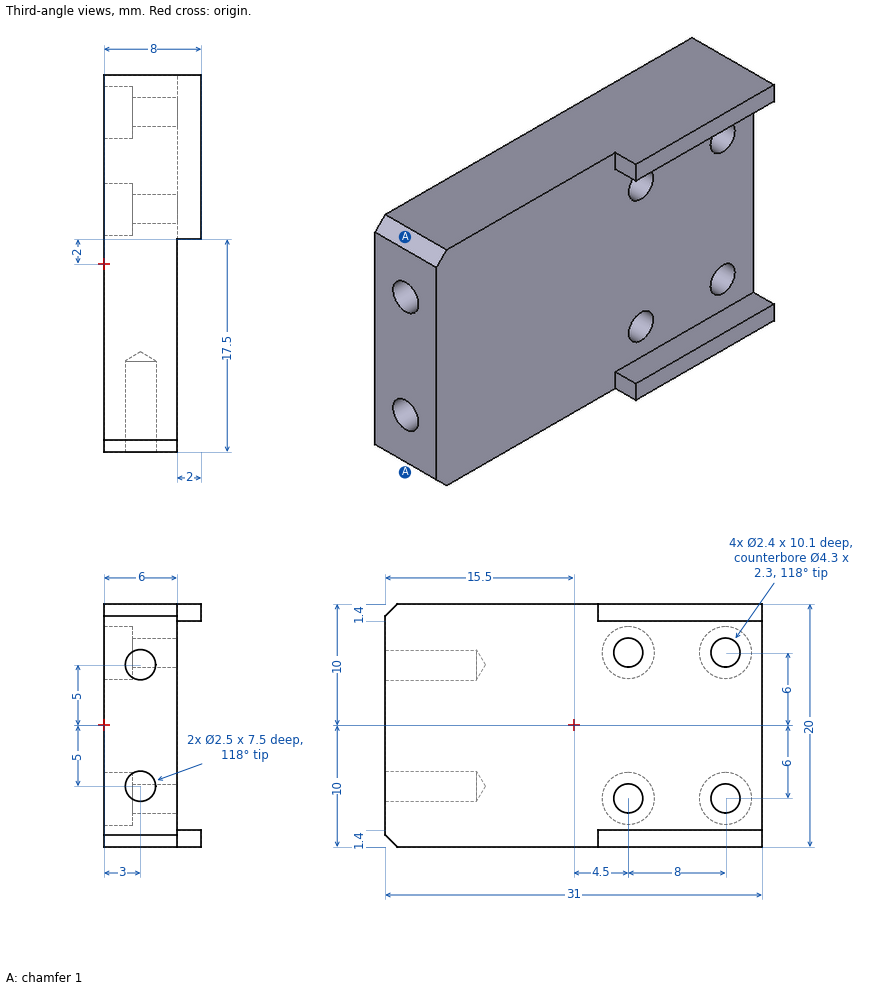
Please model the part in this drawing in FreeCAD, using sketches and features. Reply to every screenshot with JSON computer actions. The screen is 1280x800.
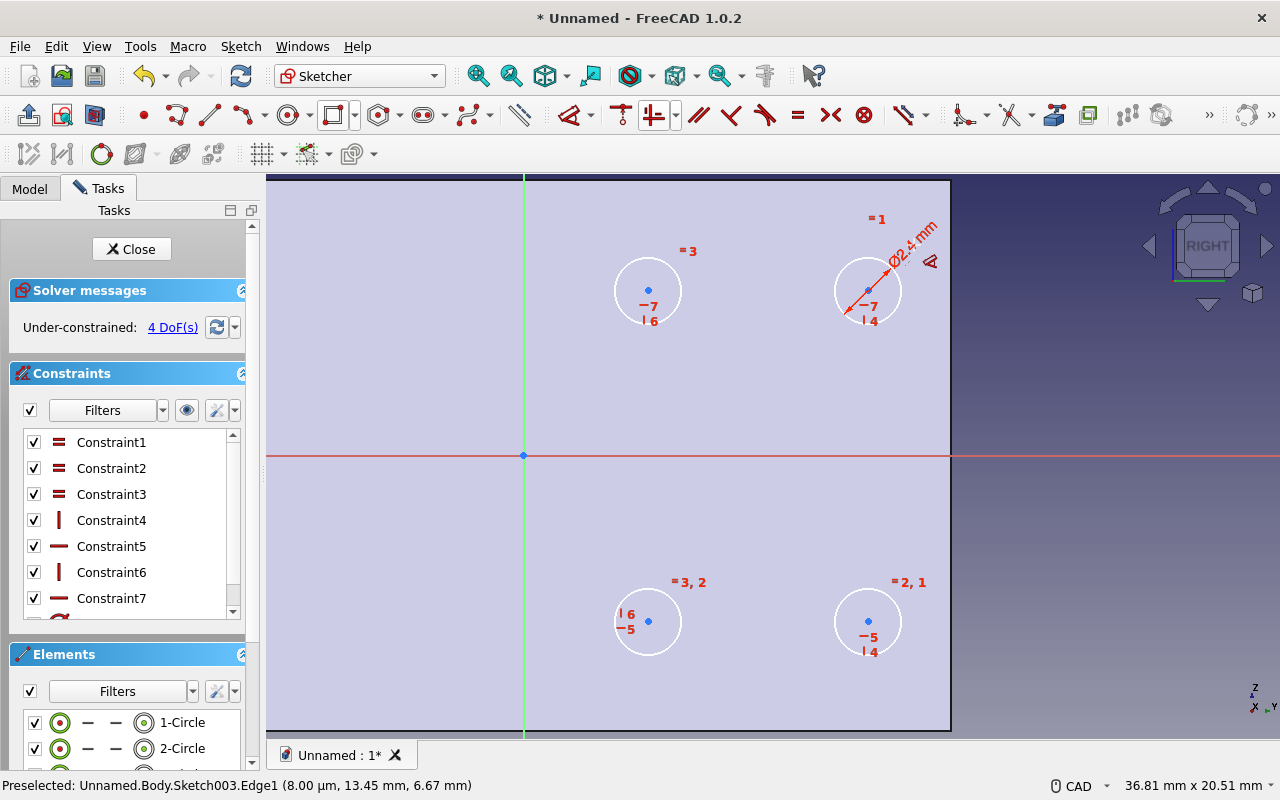
{"action": "left_click", "coordinate": [868, 291]}
{"action": "left_click", "coordinate": [490, 373]}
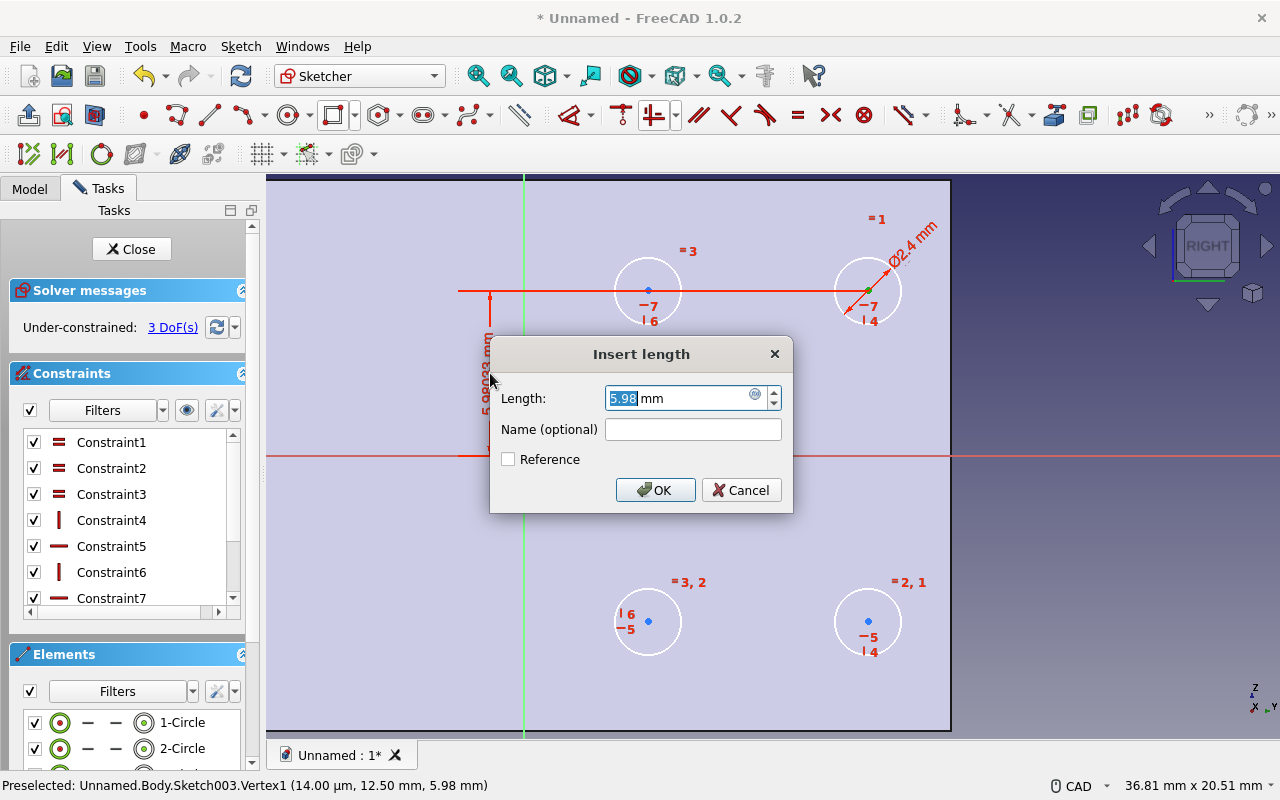
{"action": "type", "text": "6"}
{"action": "key", "text": "Return"}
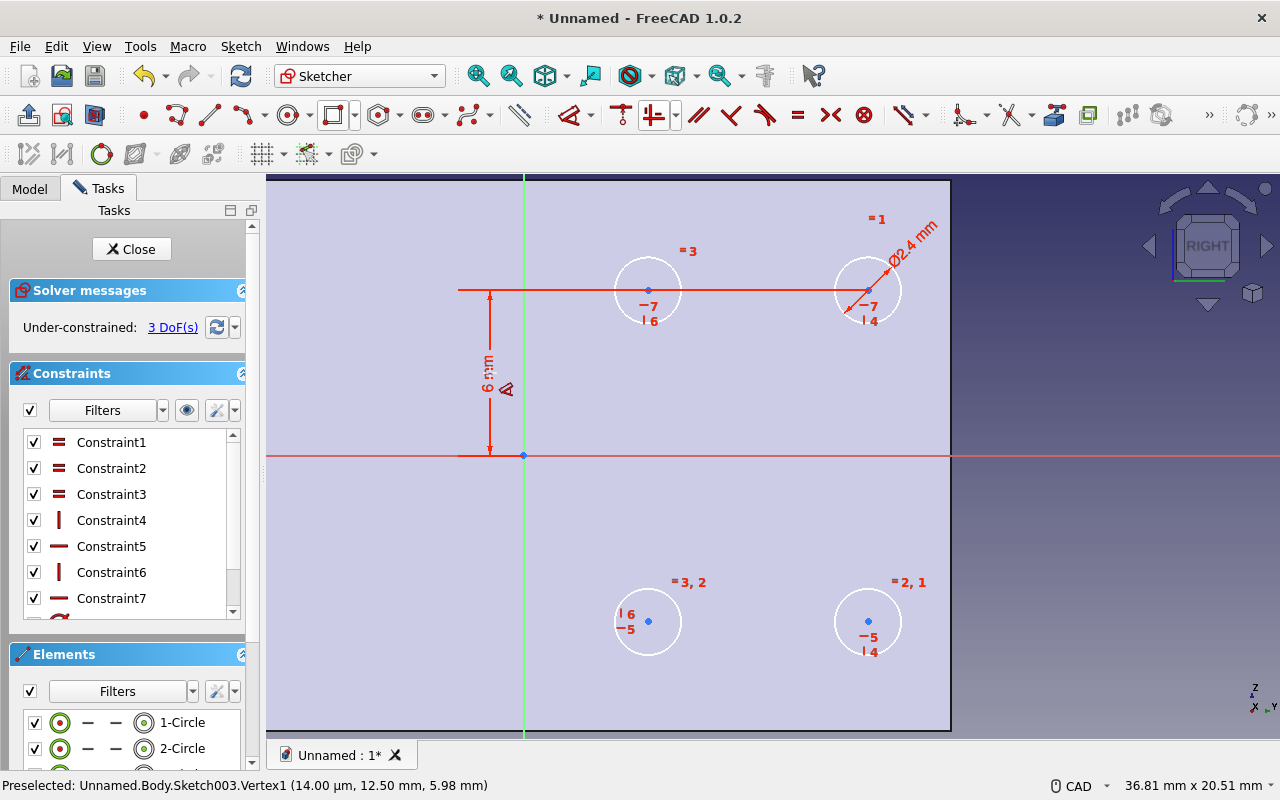
{"action": "left_click", "coordinate": [868, 622]}
{"action": "left_click", "coordinate": [490, 539]}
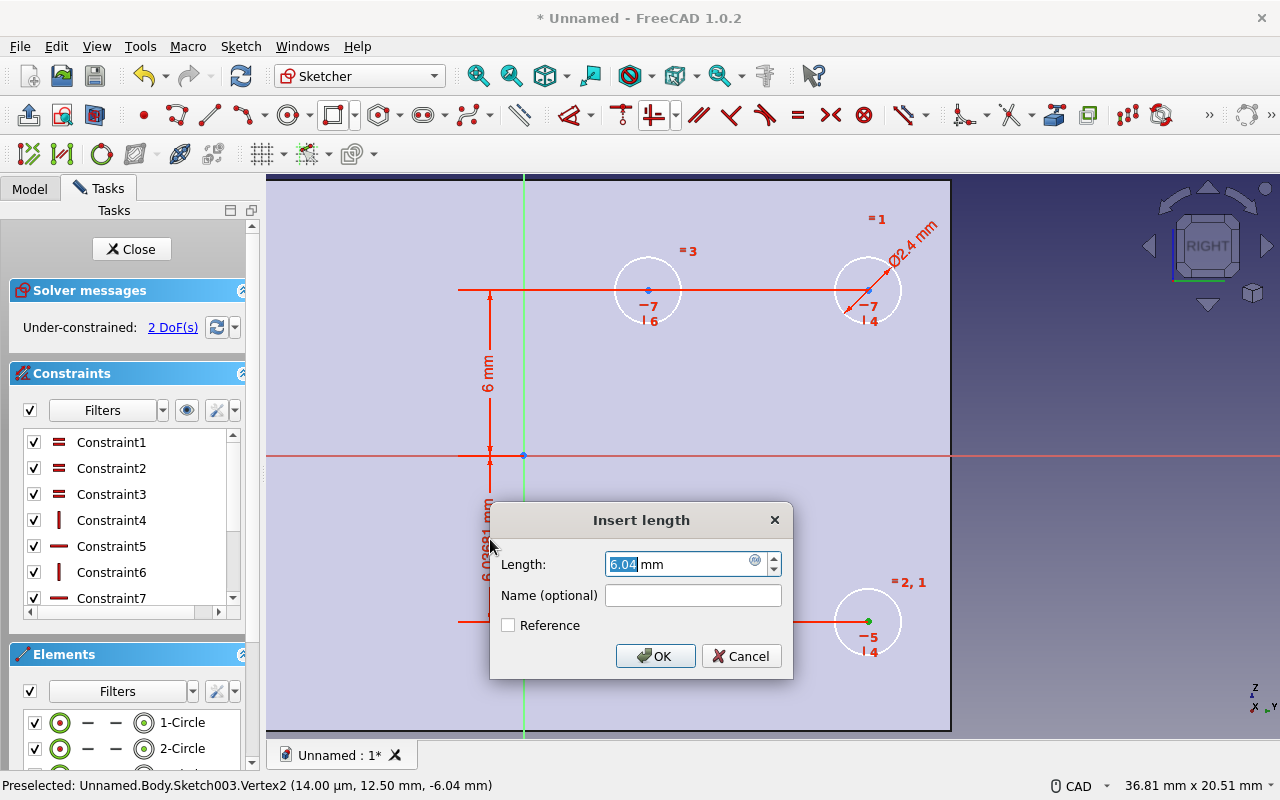
{"action": "type", "text": "6"}
{"action": "key", "text": "Return"}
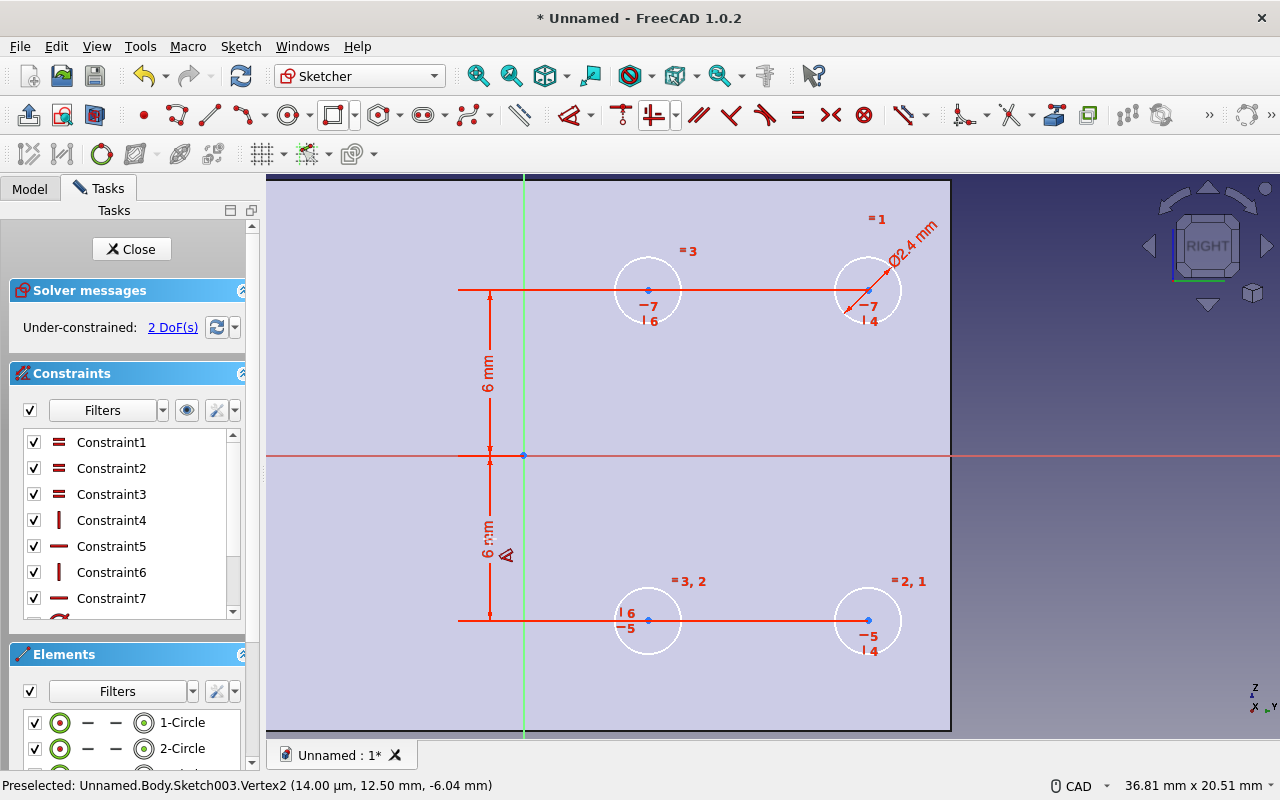
{"action": "left_click", "coordinate": [868, 621]}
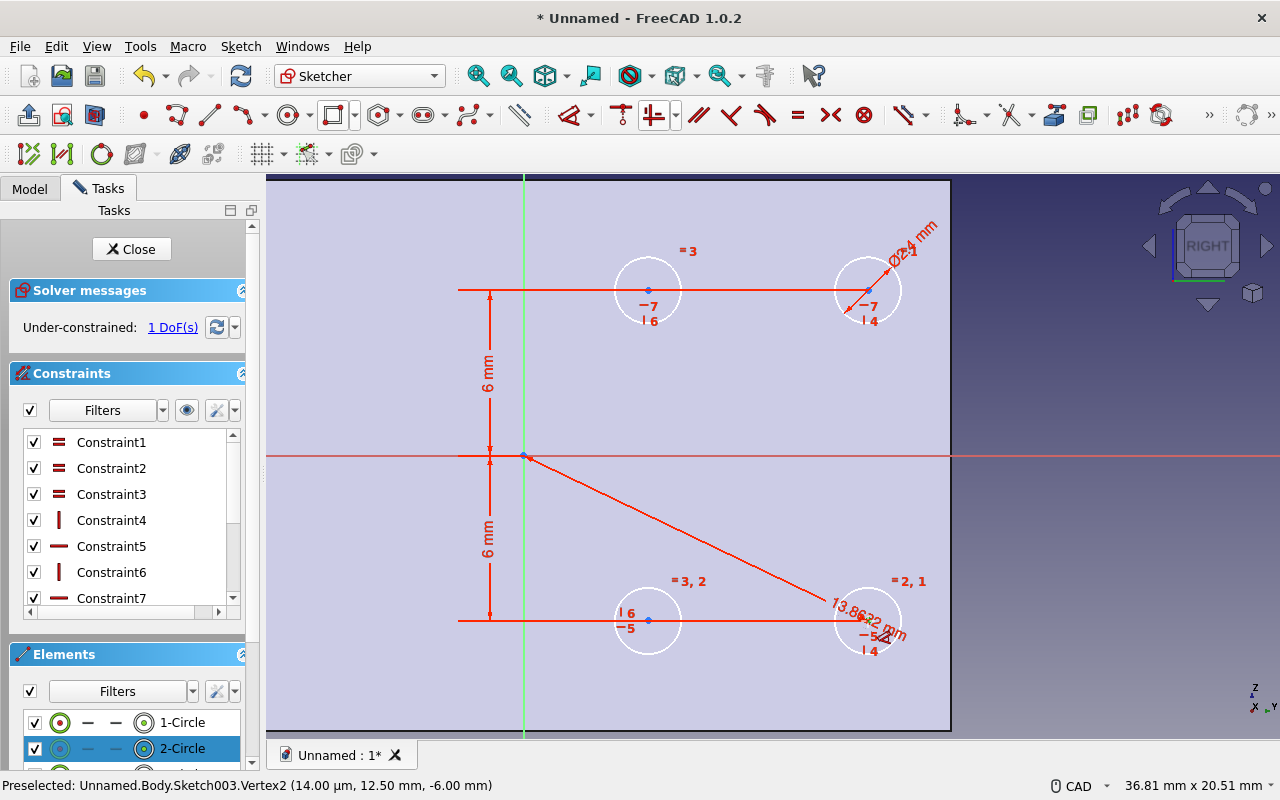
{"action": "left_click", "coordinate": [648, 621]}
{"action": "left_click", "coordinate": [758, 655]}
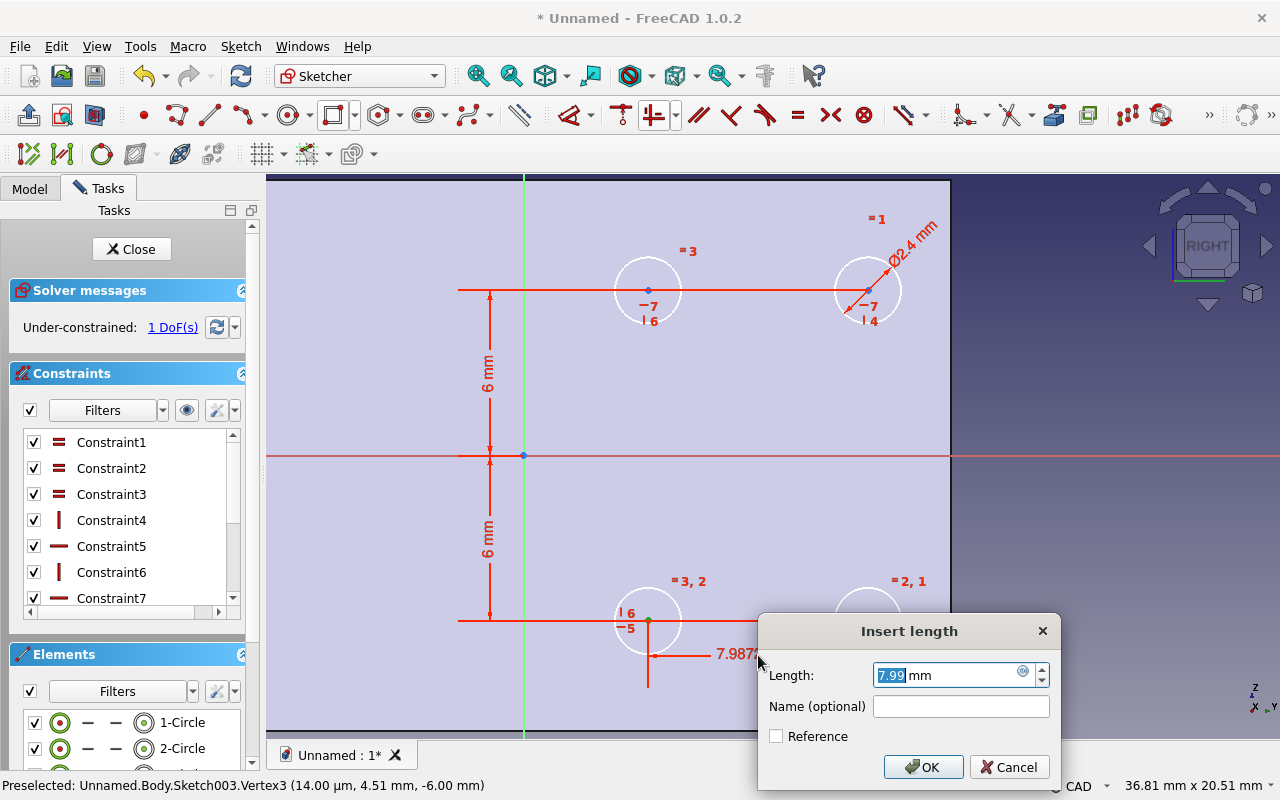
{"action": "type", "text": "8"}
{"action": "key", "text": "Return"}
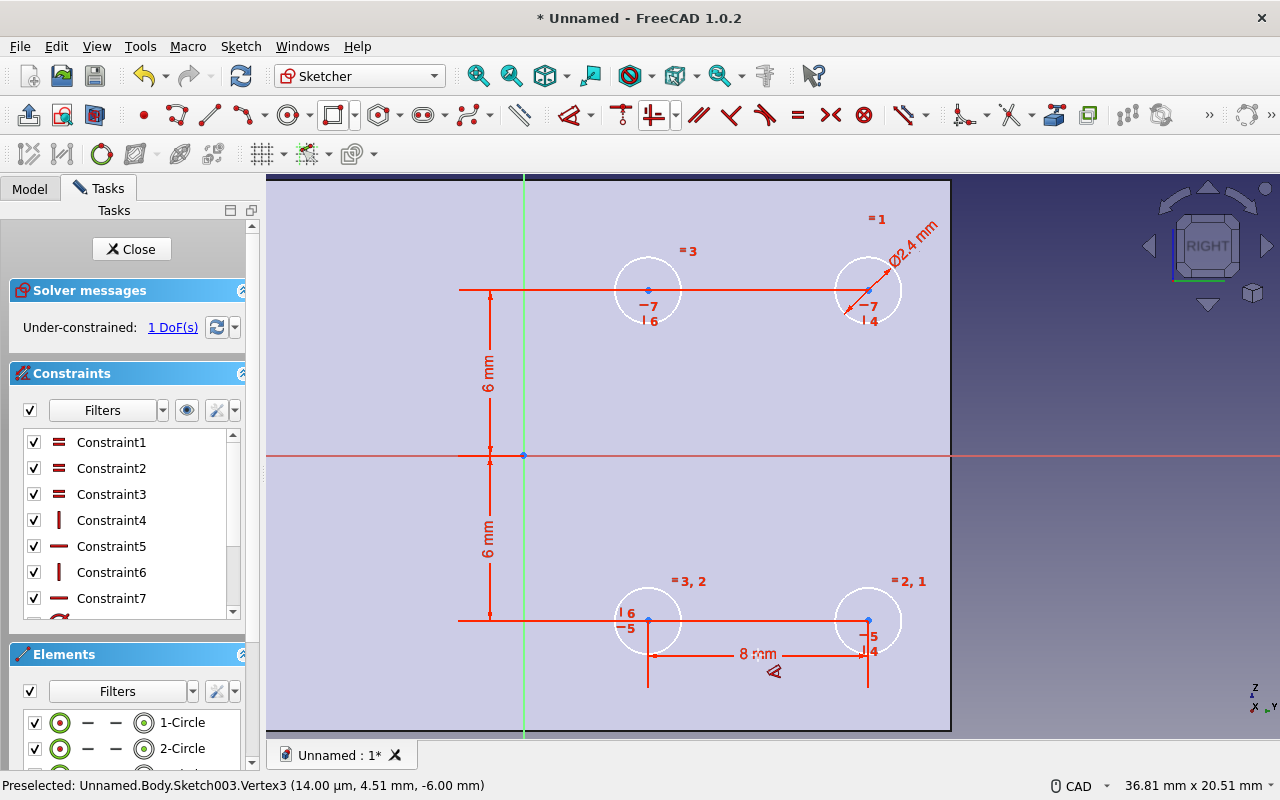
{"action": "left_click", "coordinate": [648, 621]}
{"action": "left_click", "coordinate": [586, 655]}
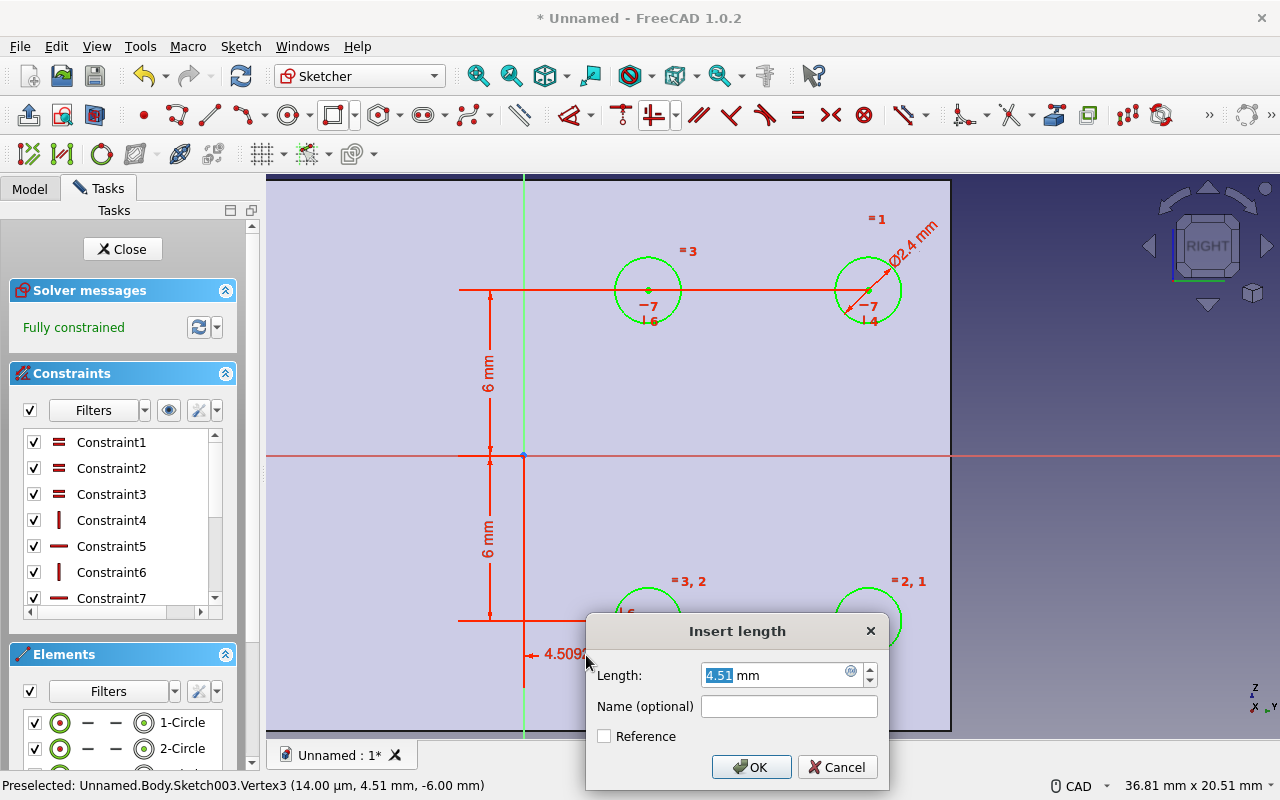
{"action": "type", "text": "4.5"}
{"action": "key", "text": "Return"}
{"action": "key", "text": "Escape"}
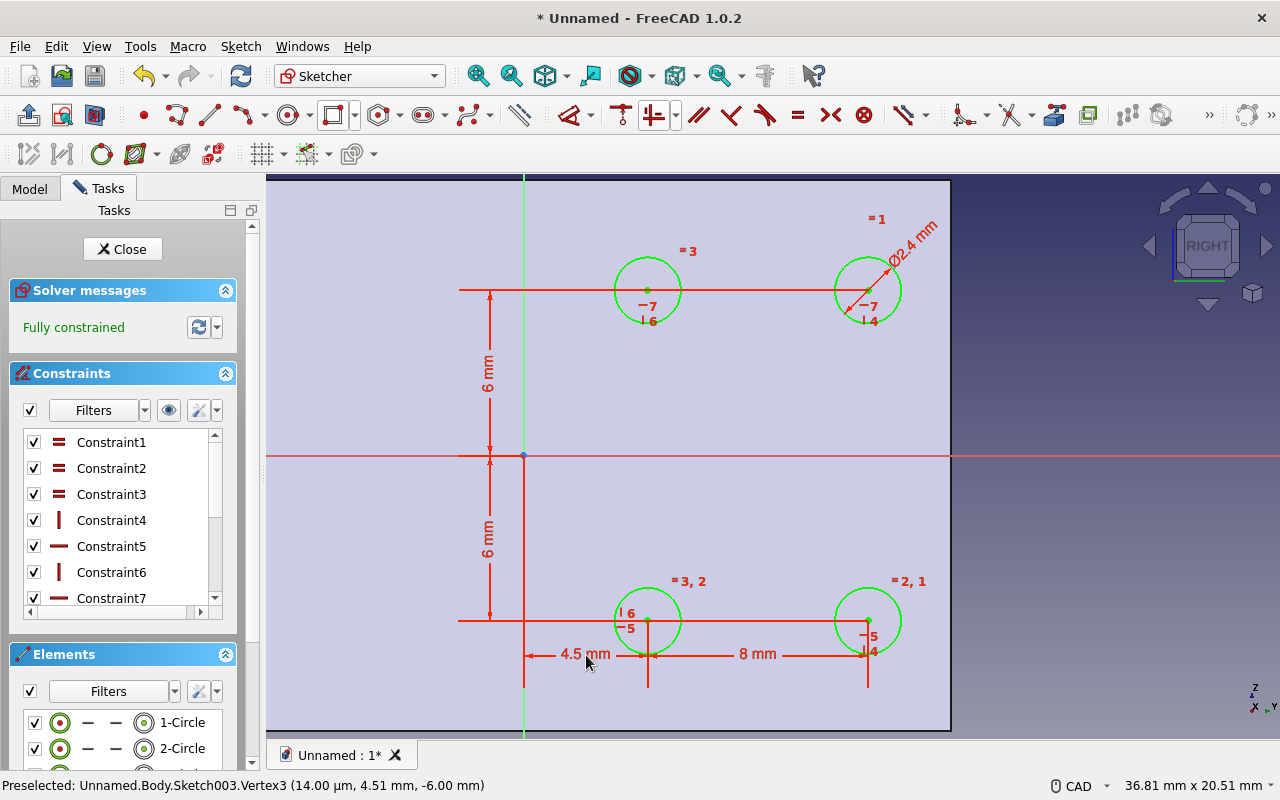
{"action": "left_click", "coordinate": [123, 249]}